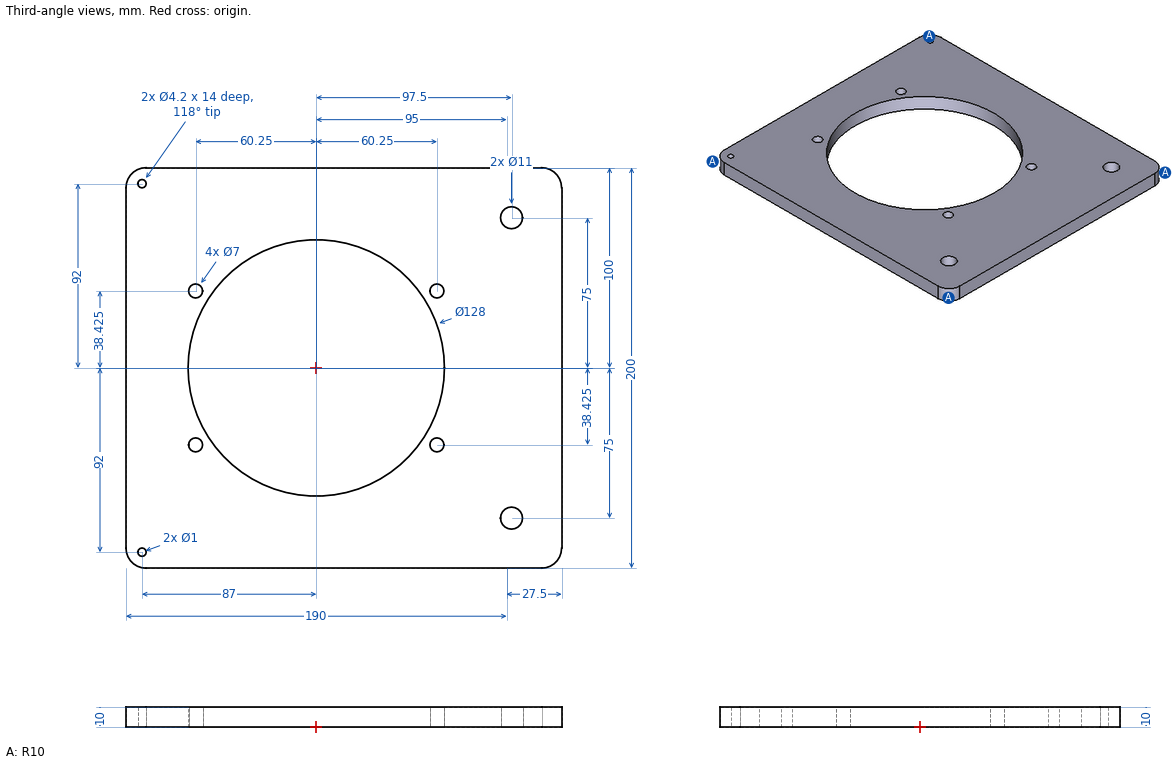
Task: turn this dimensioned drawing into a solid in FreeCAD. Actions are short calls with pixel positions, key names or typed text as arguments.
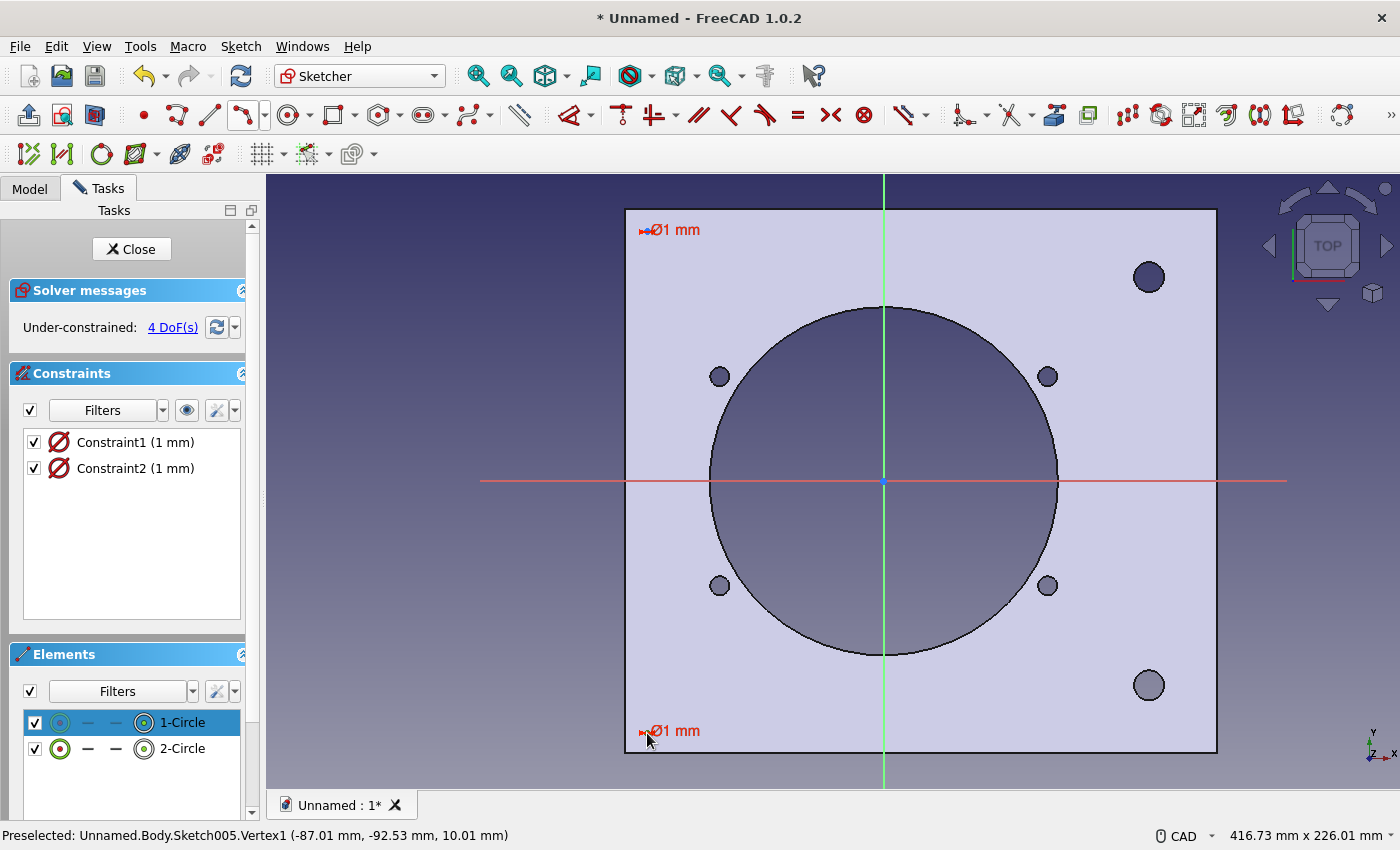
click(647, 232)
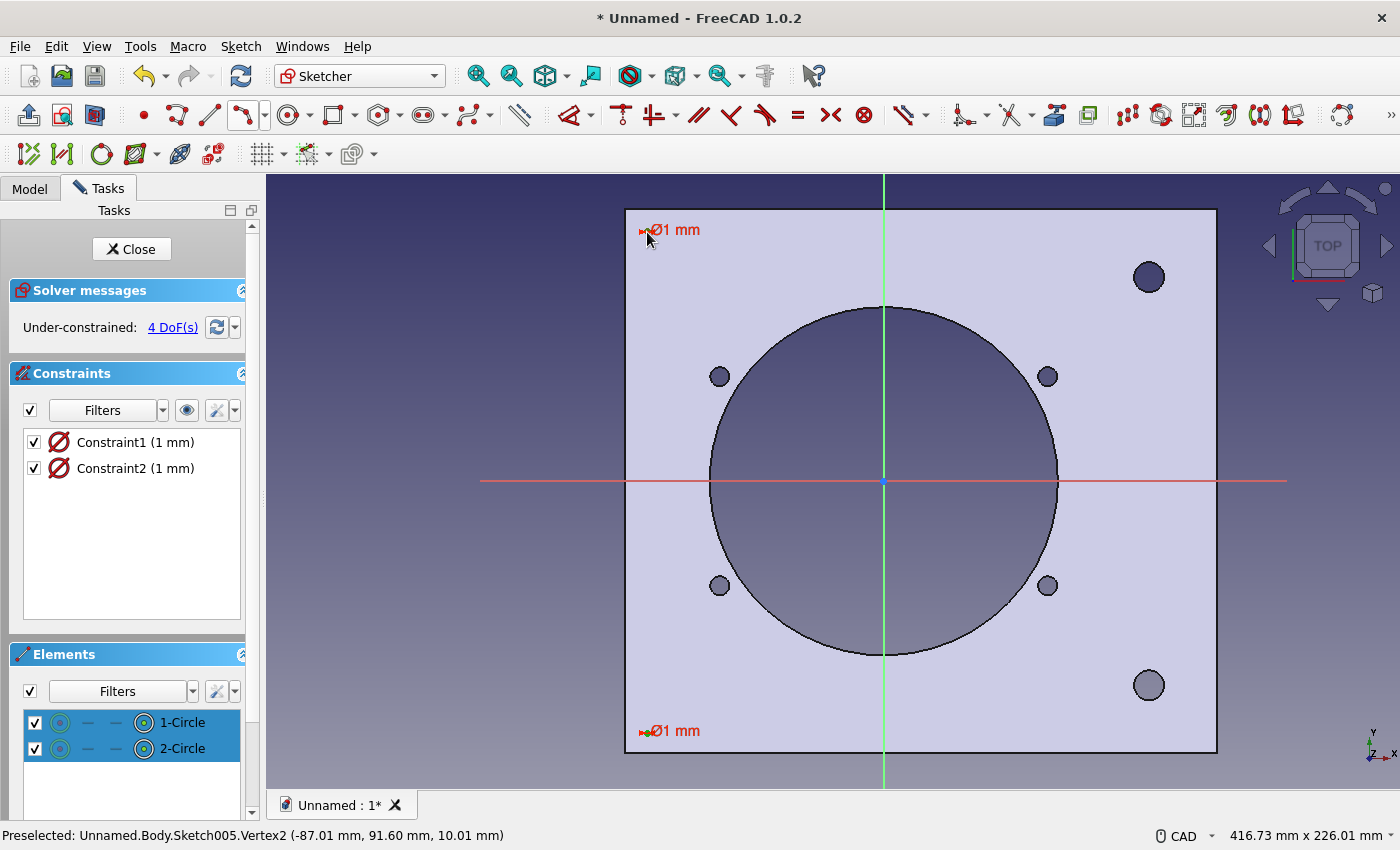
key(v)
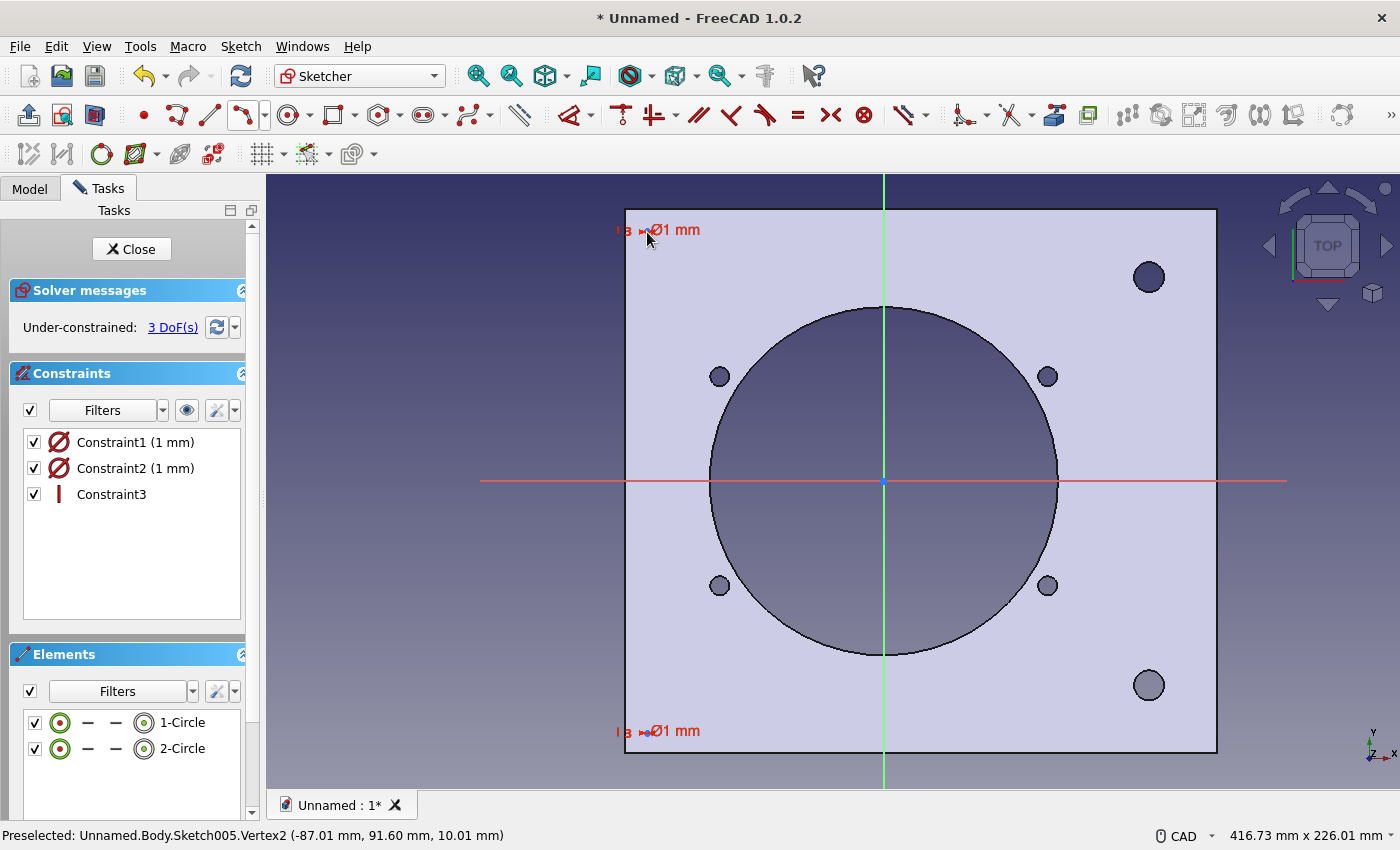
key(d)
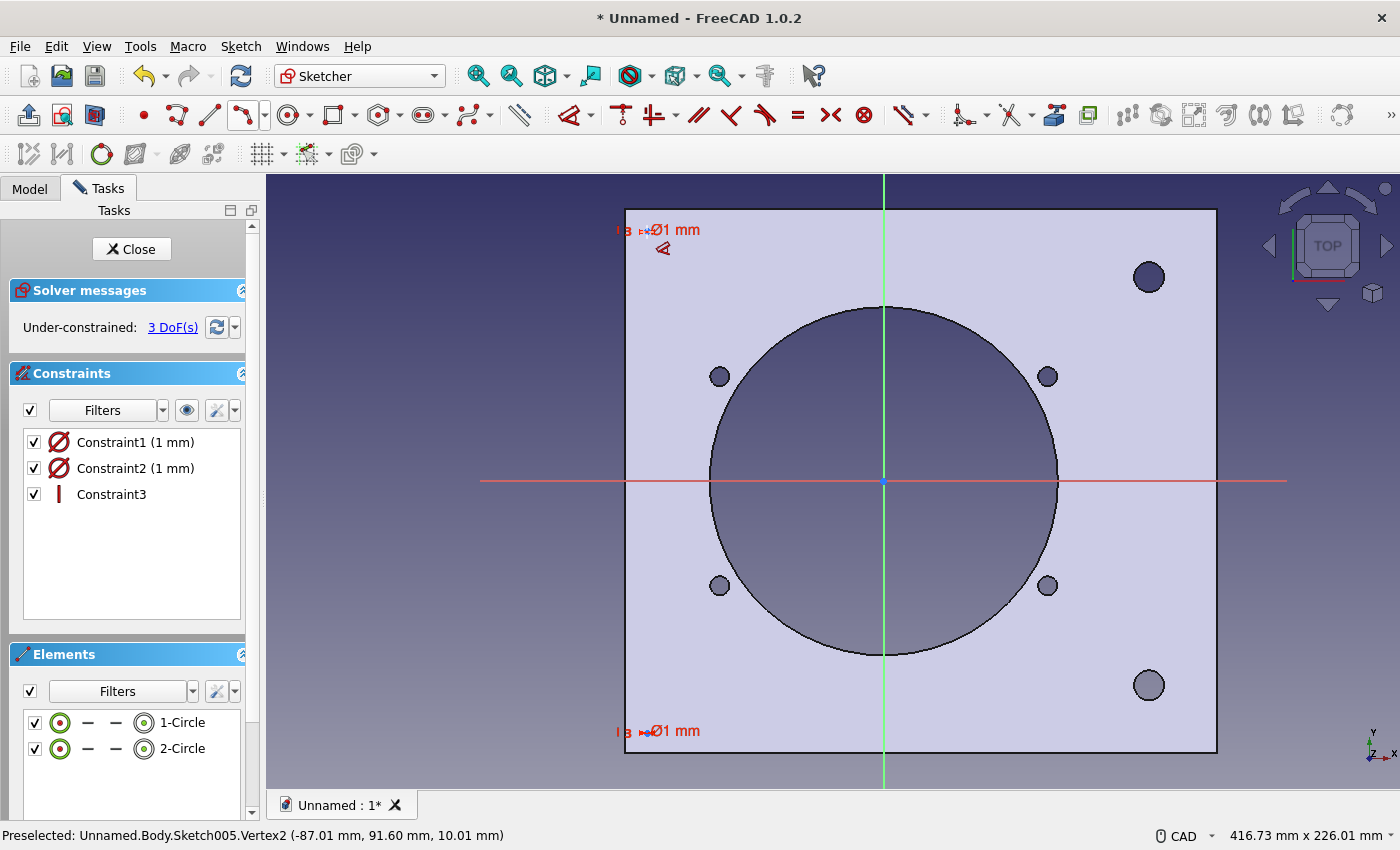
click(647, 733)
click(765, 447)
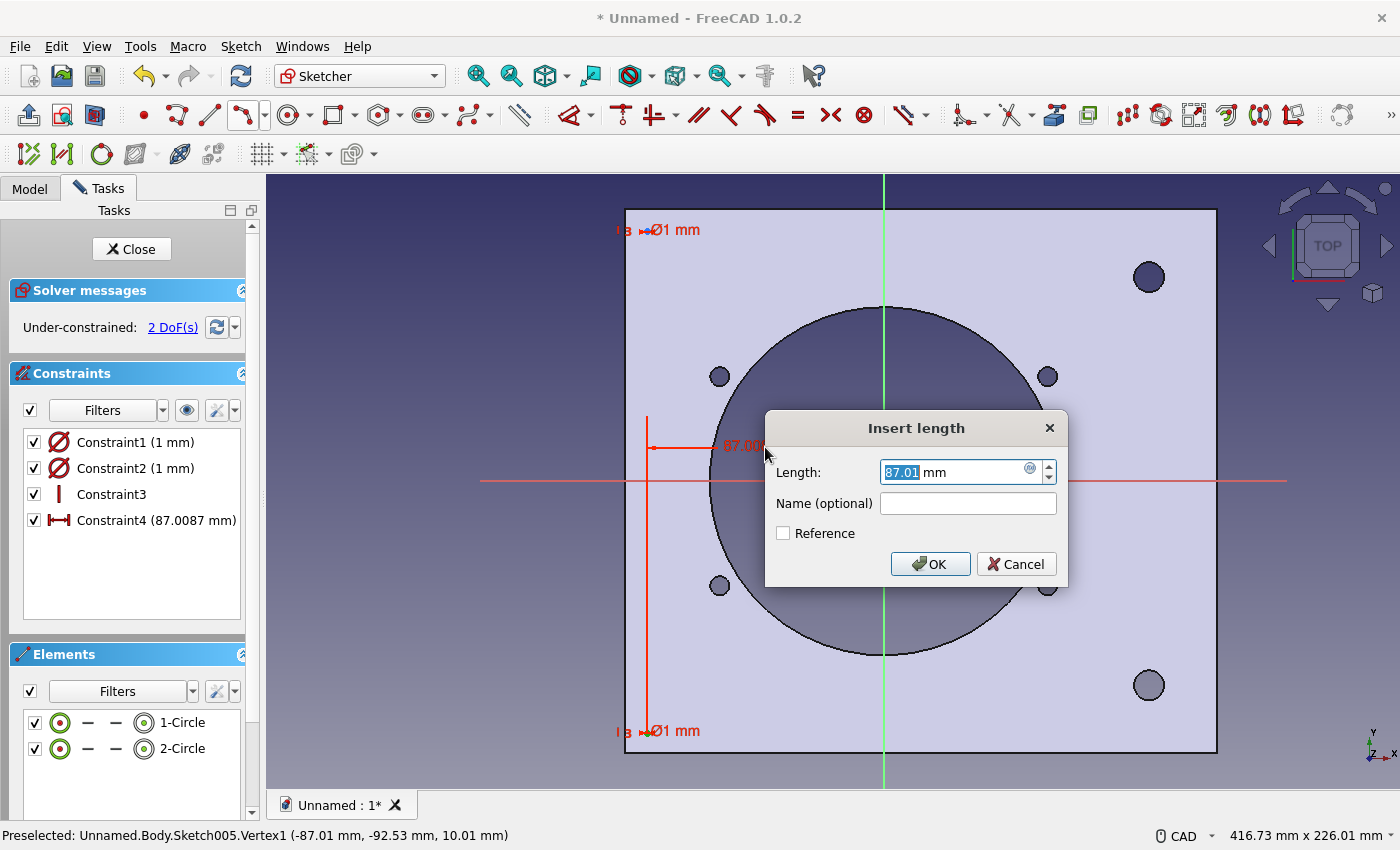
text(87)
key(Return)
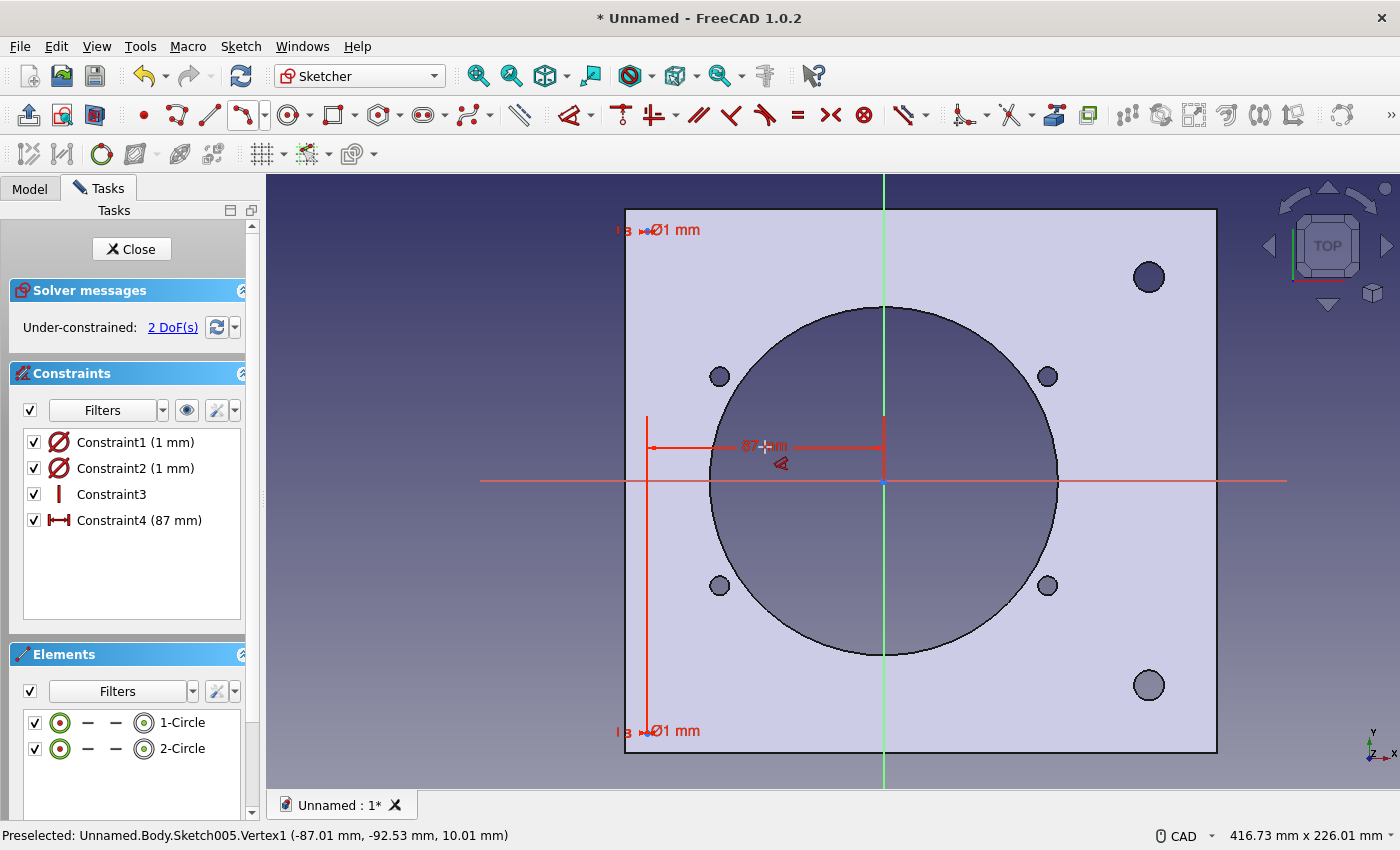
click(647, 733)
click(918, 607)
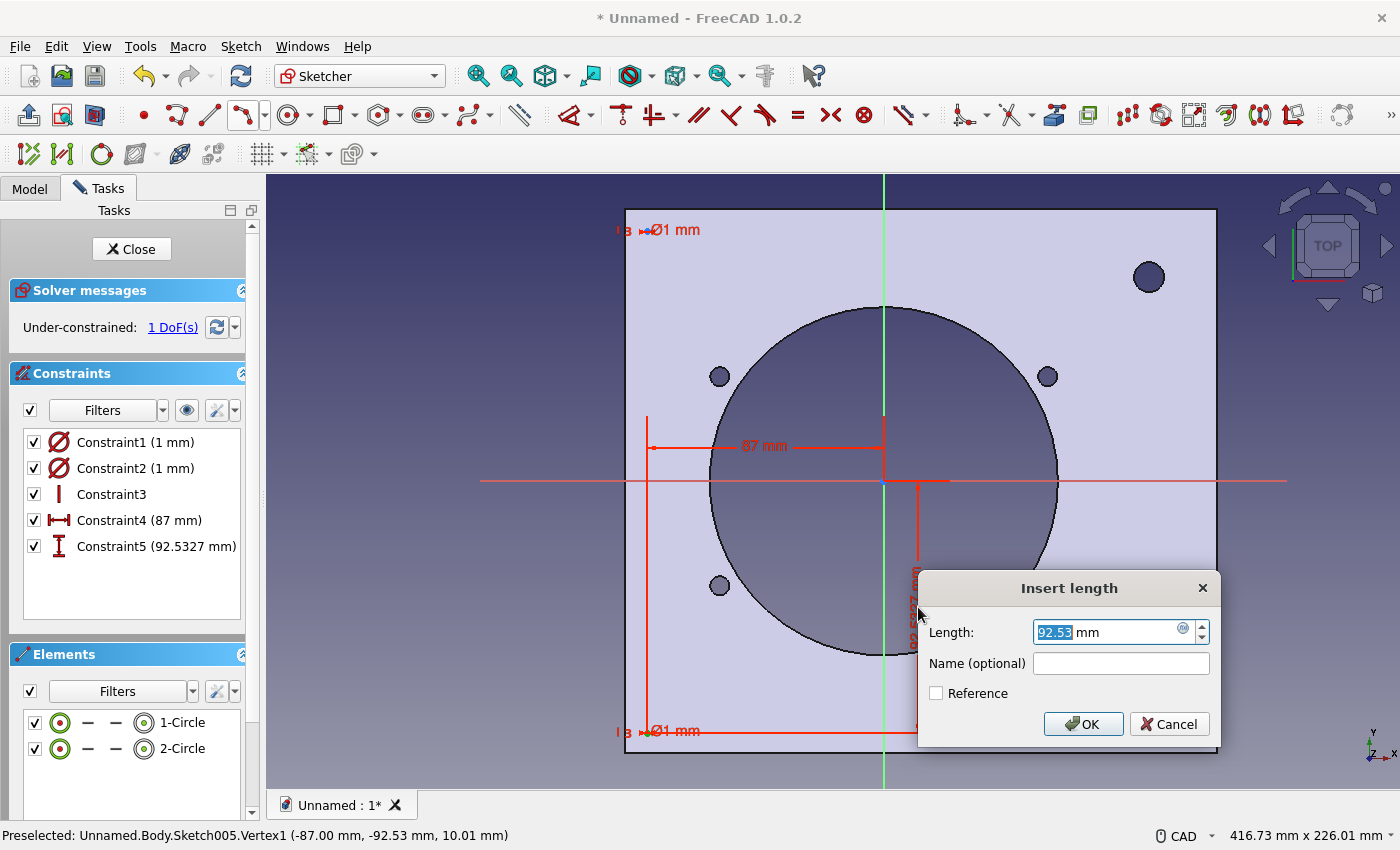
text(92)
key(Return)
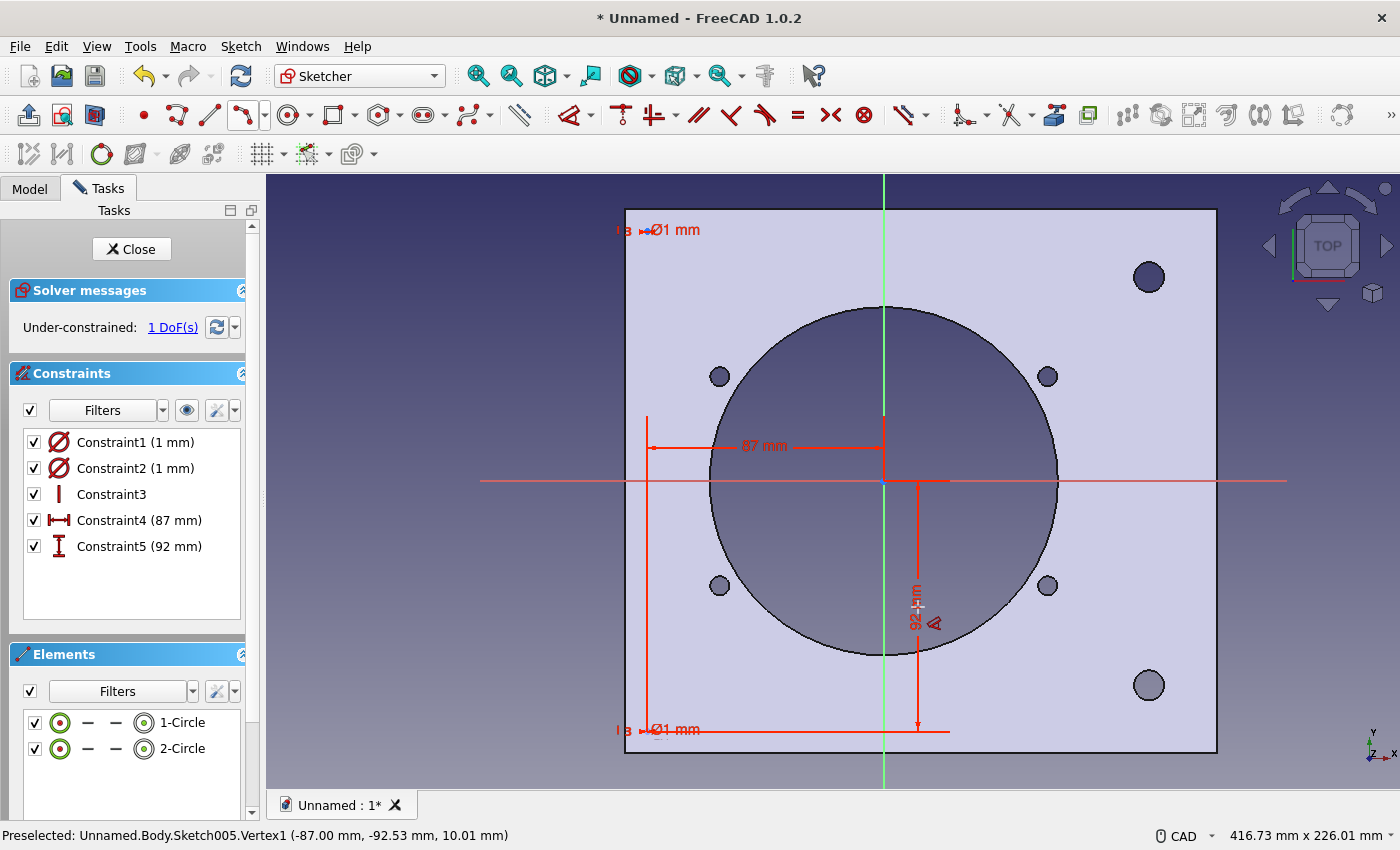
click(647, 232)
click(918, 357)